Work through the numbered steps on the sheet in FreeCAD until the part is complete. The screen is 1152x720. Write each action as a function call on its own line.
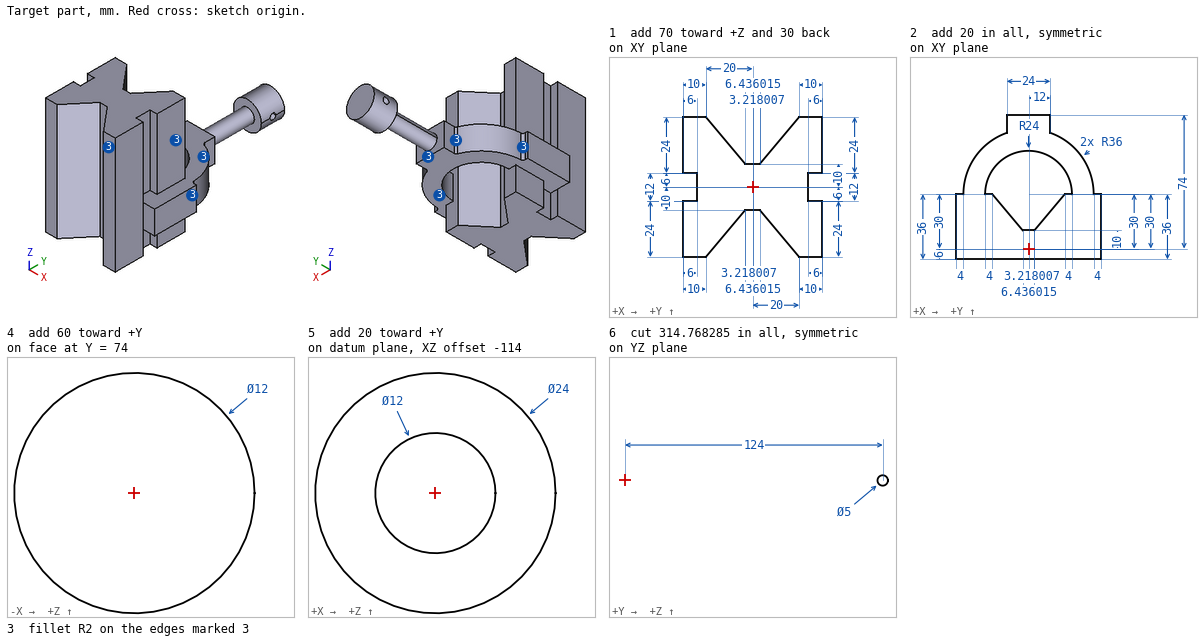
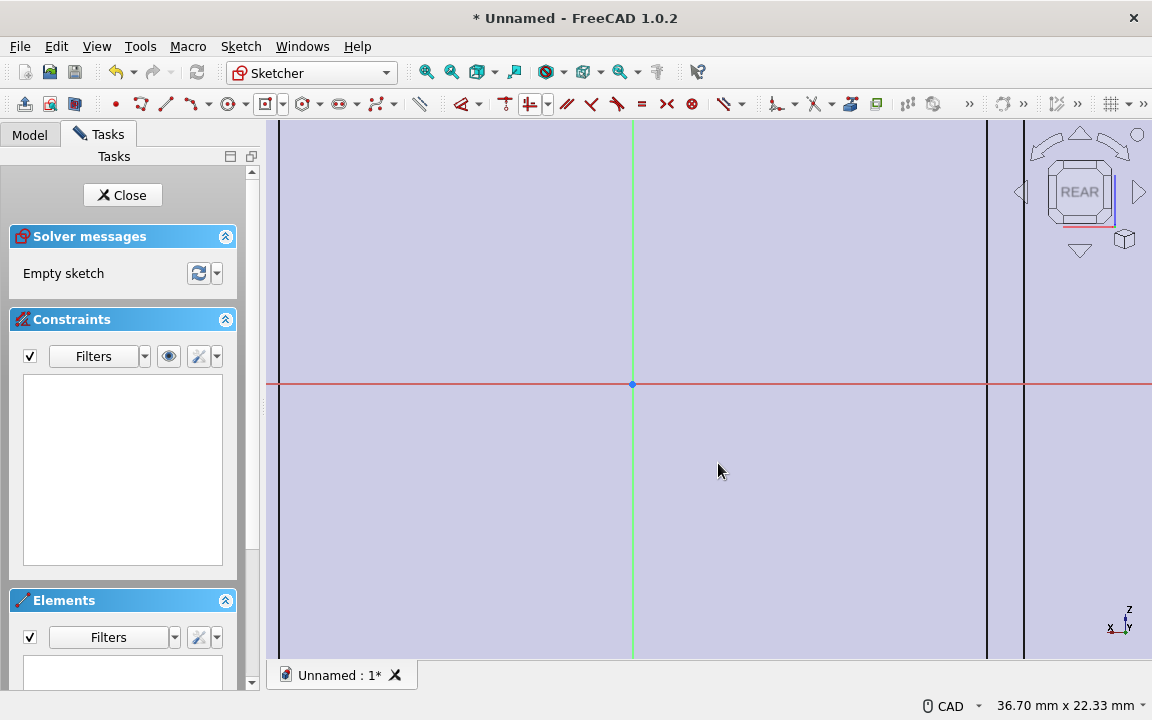
click(228, 104)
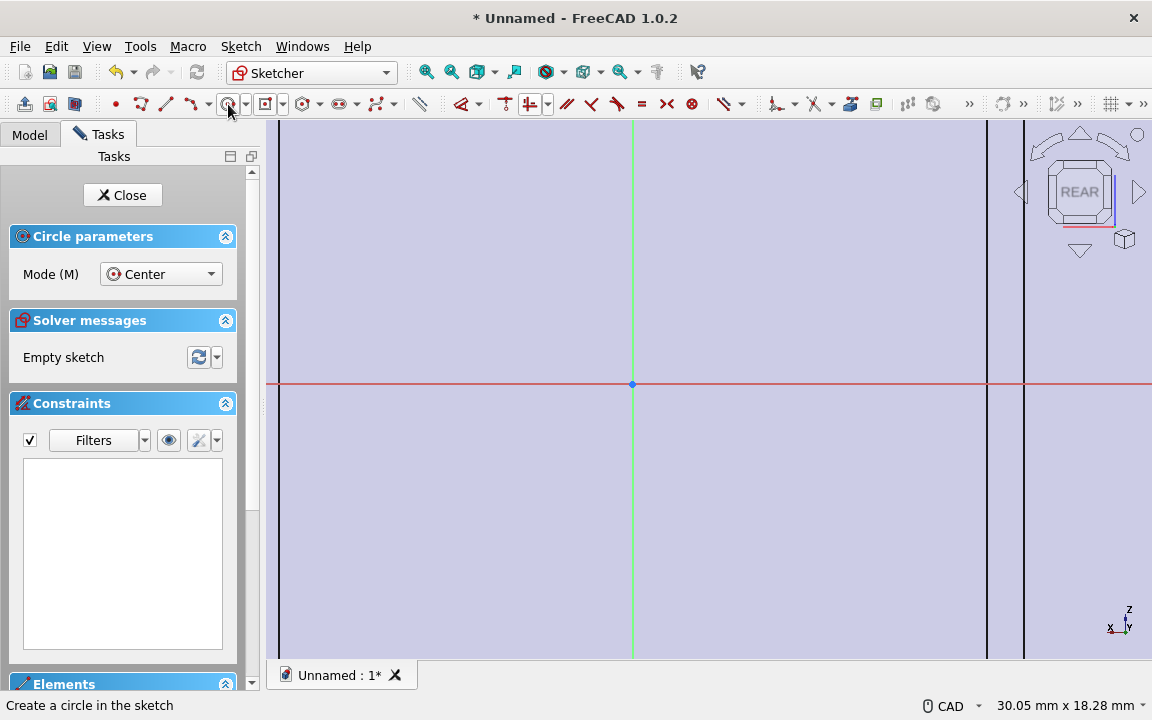
click(633, 384)
move(758, 259)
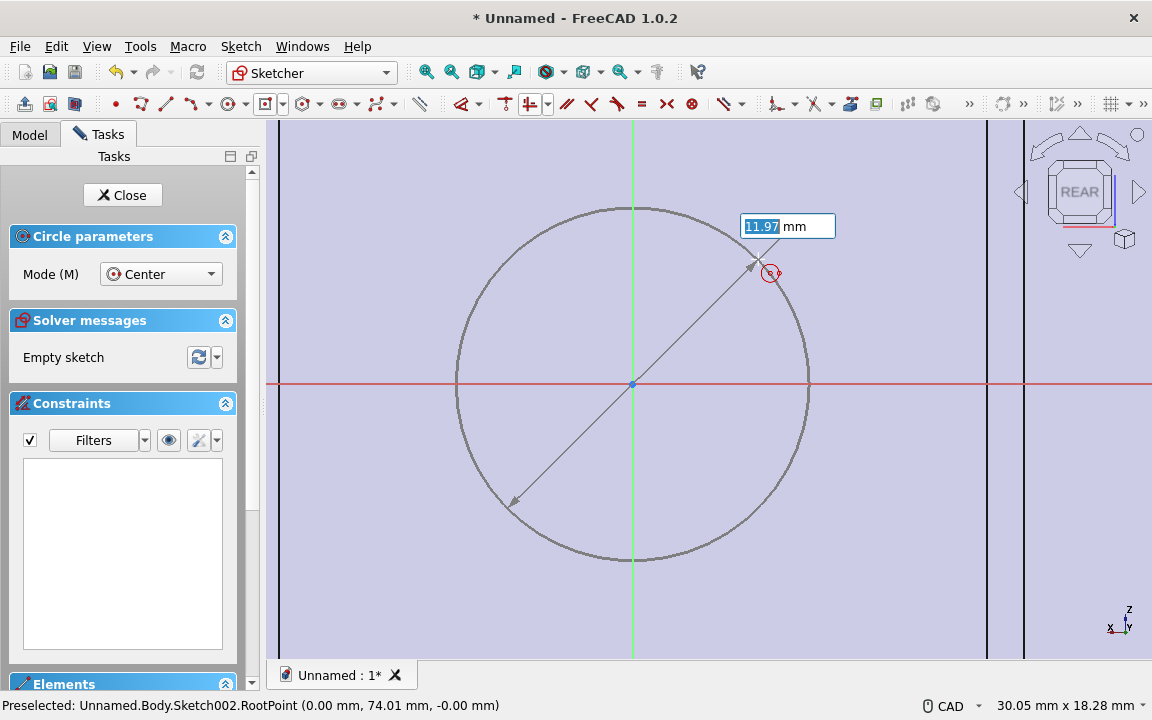
text(12)
key(Return)
key(Escape)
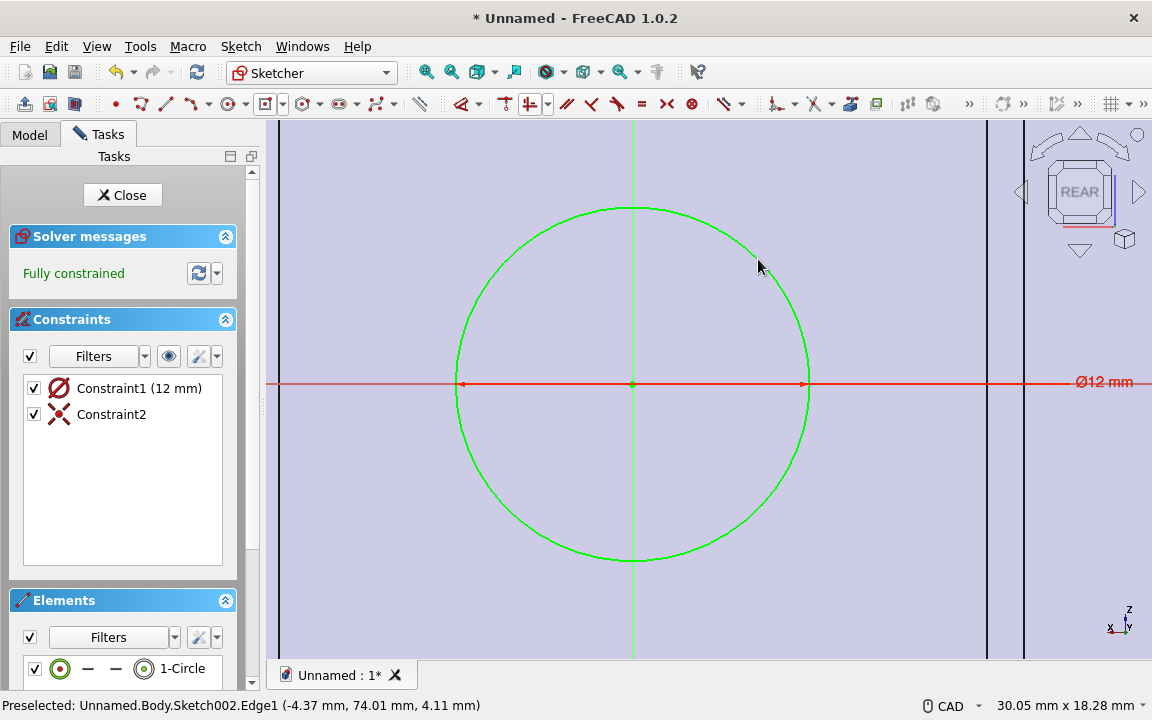
click(123, 195)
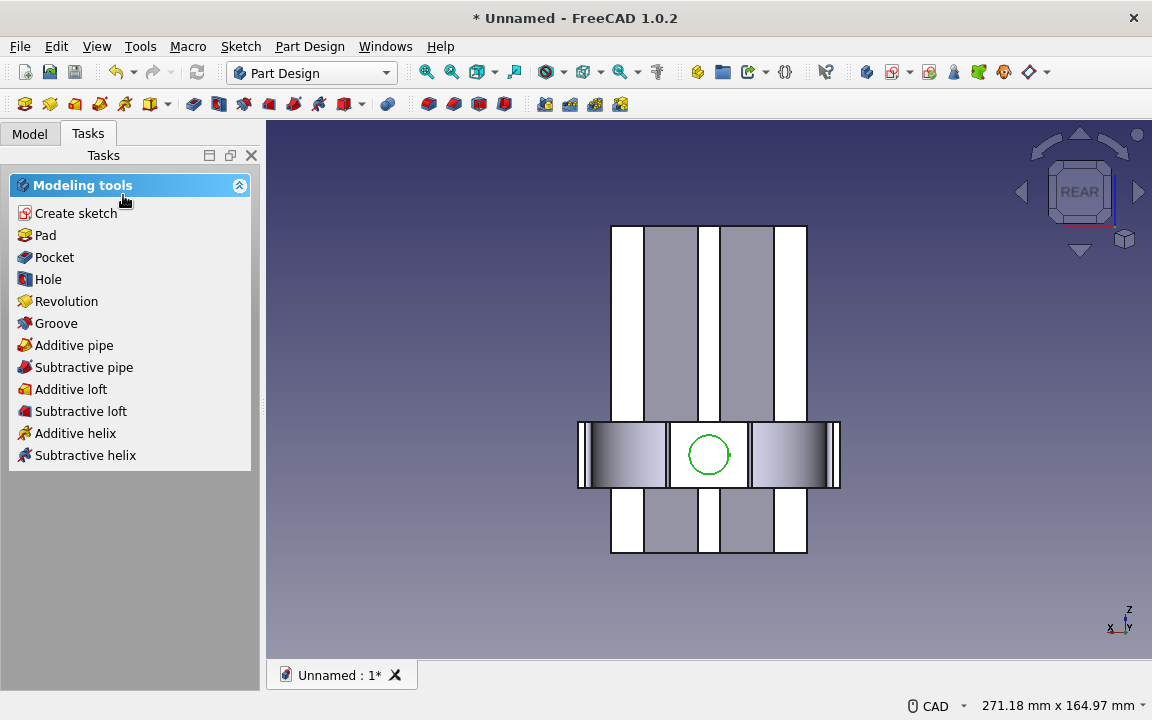
click(25, 104)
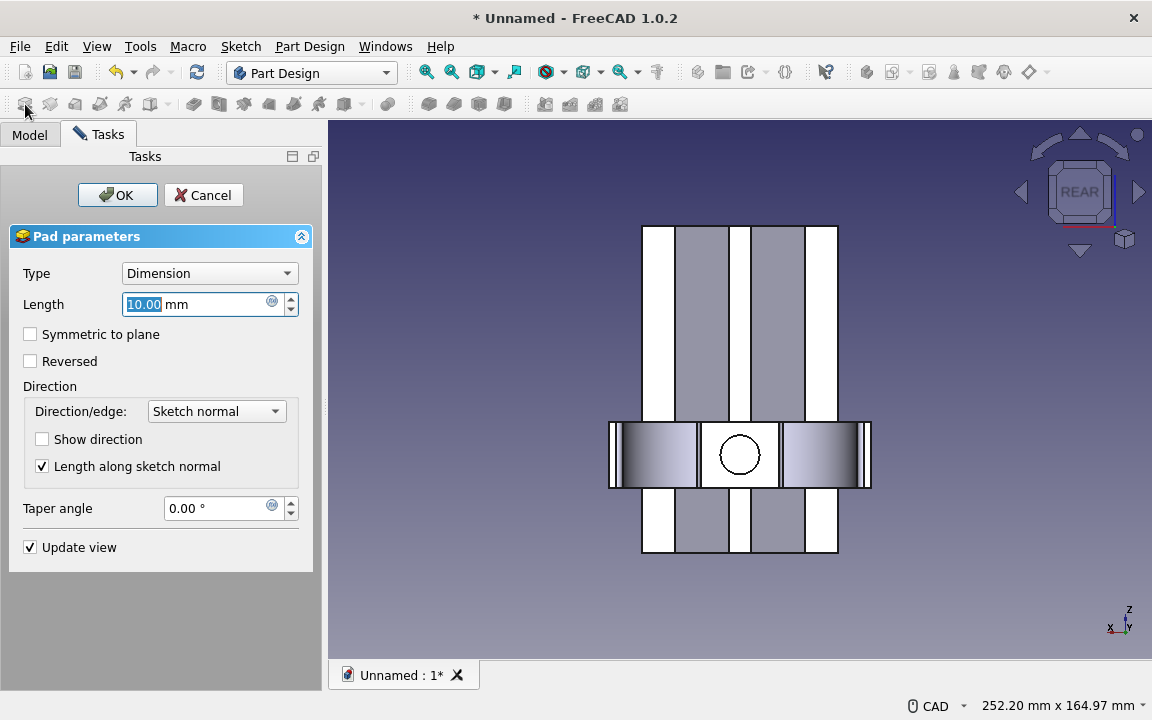
text(60)
key(Tab)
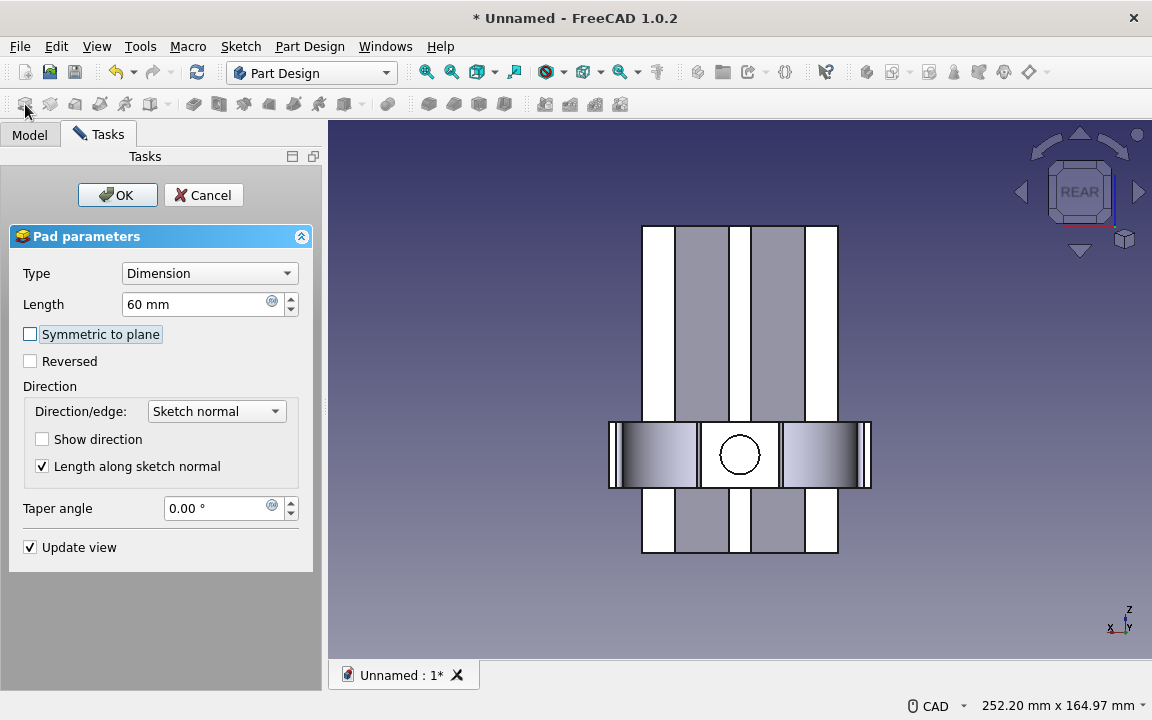
click(118, 195)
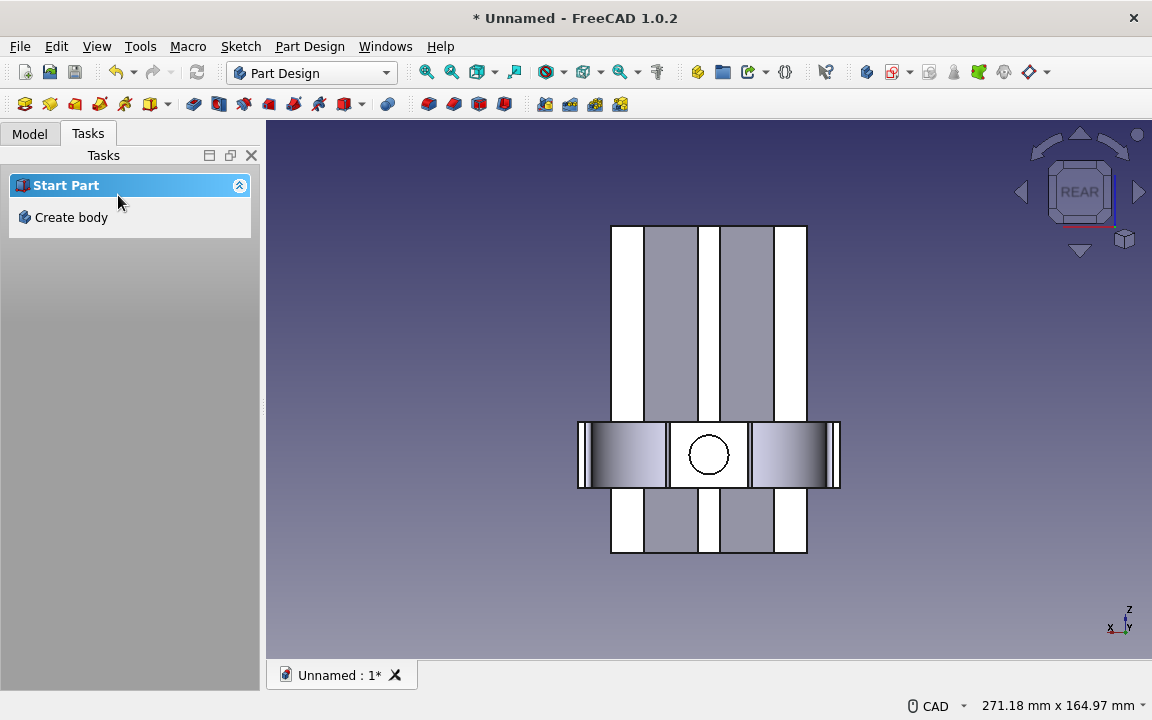
click(30, 134)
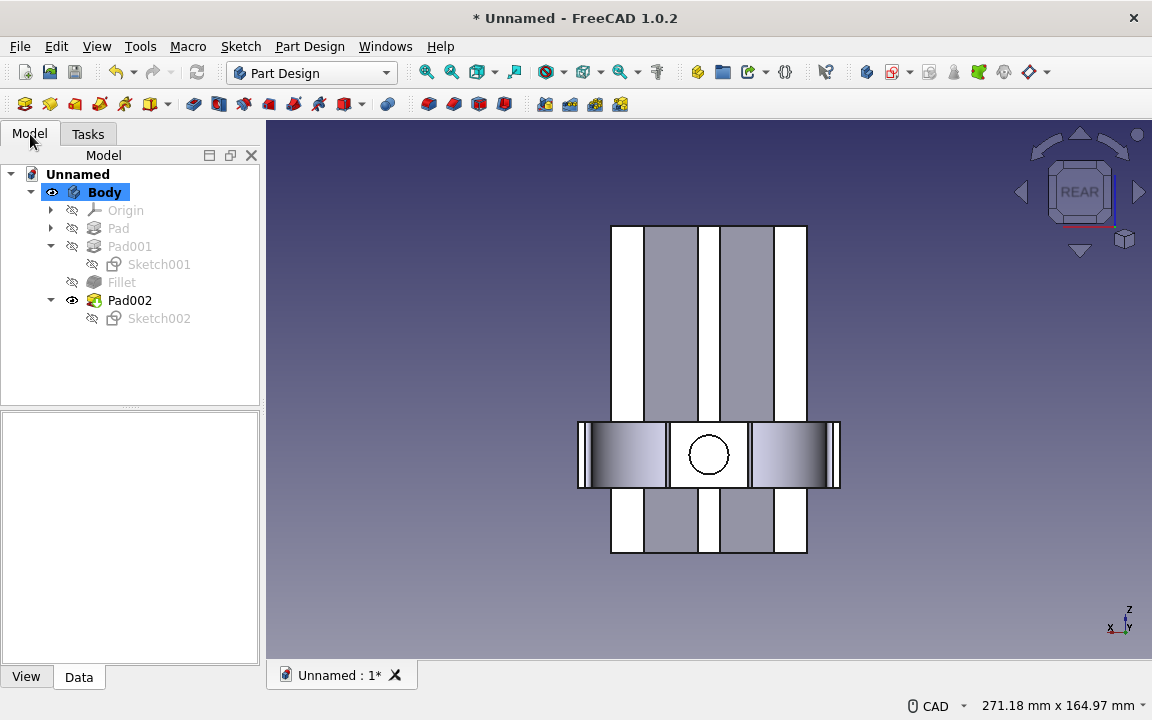
click(51, 210)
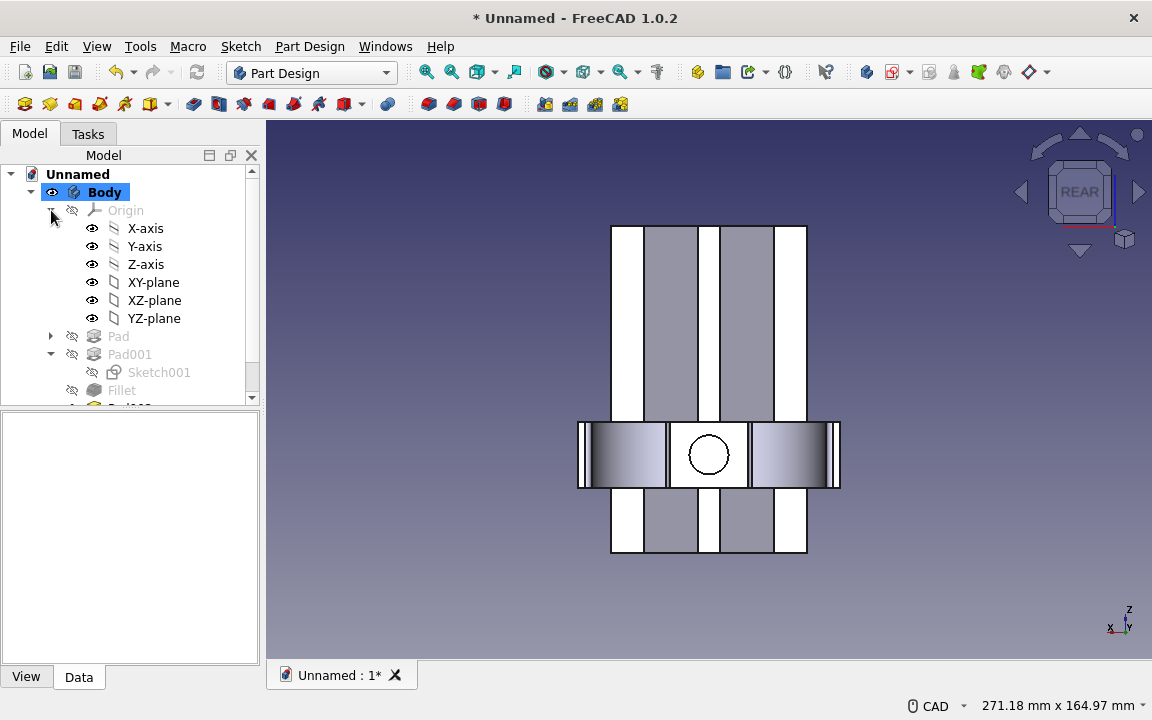
click(137, 300)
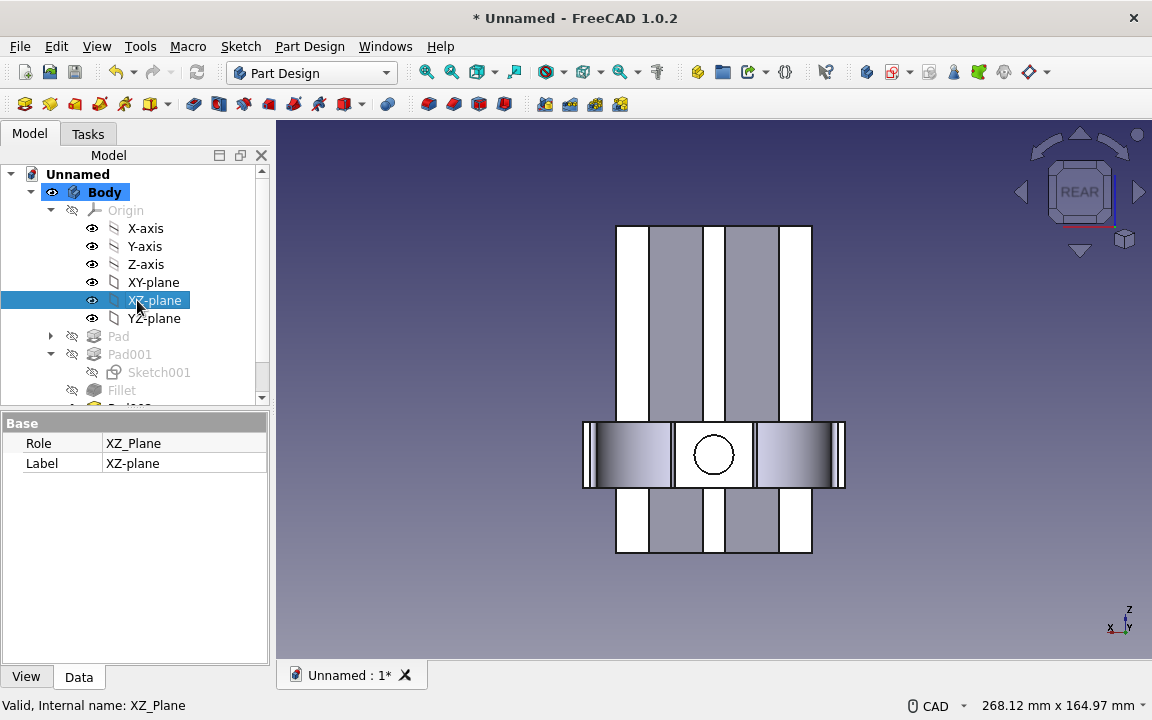
click(1028, 72)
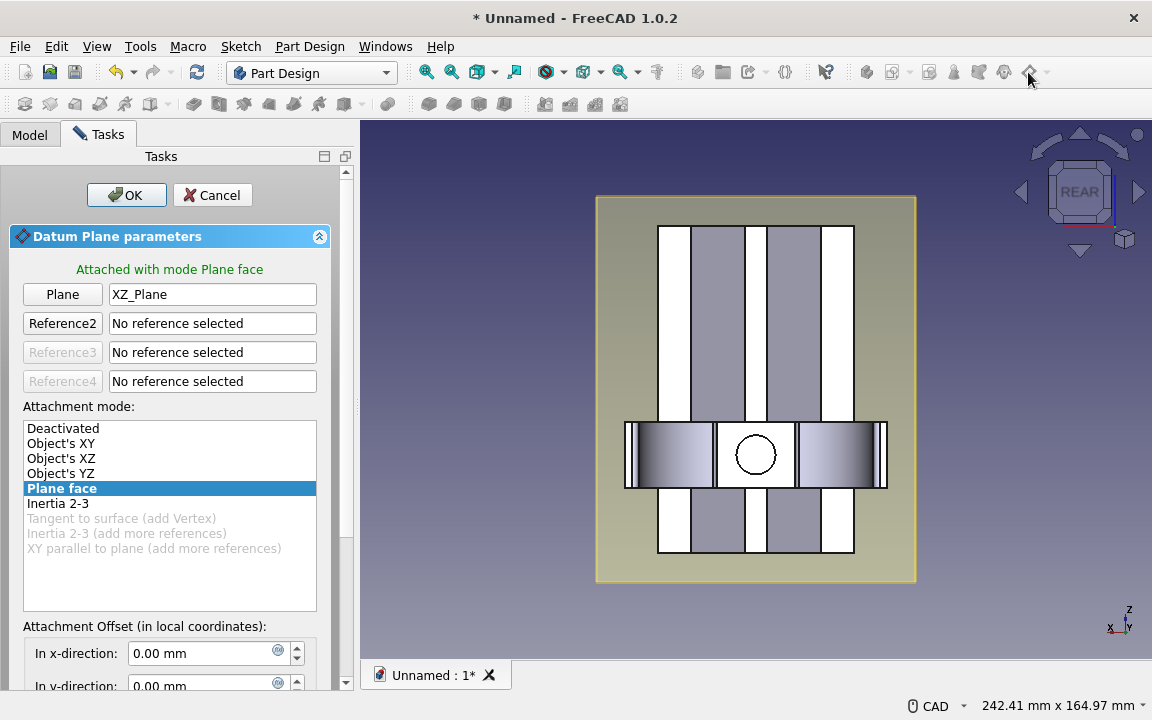
scroll(346, 428, down, 2)